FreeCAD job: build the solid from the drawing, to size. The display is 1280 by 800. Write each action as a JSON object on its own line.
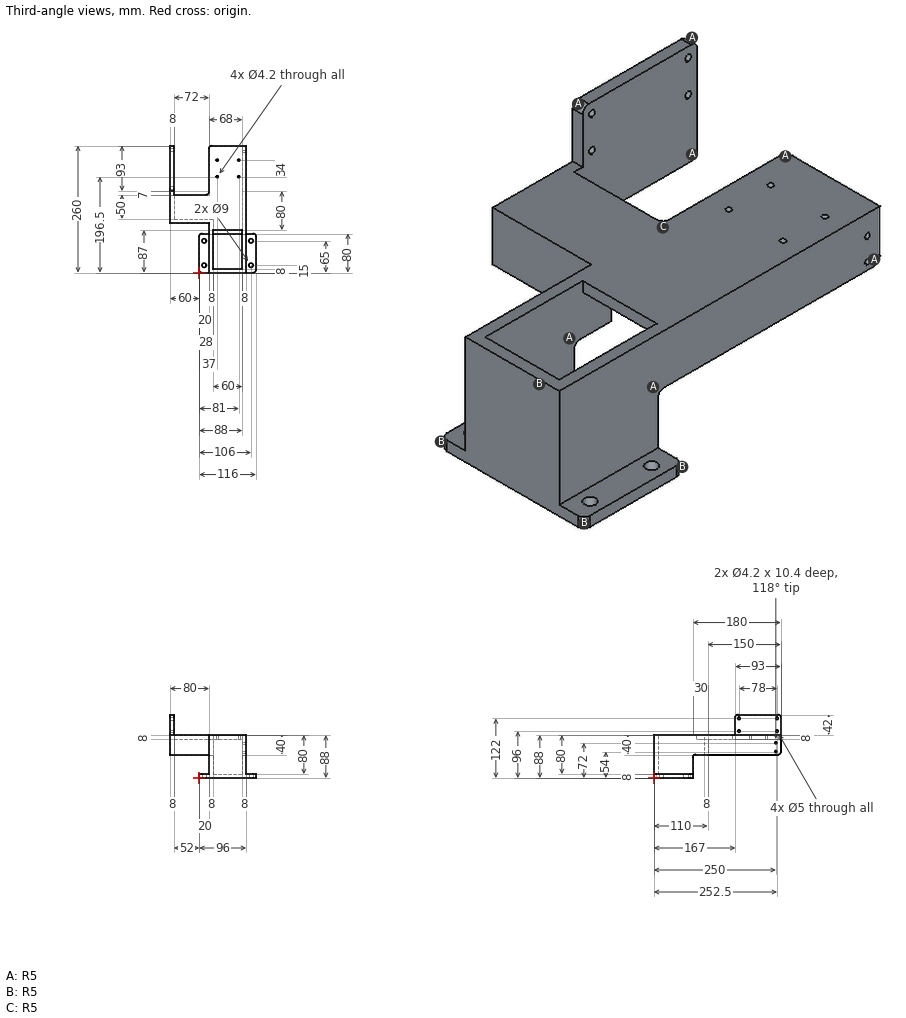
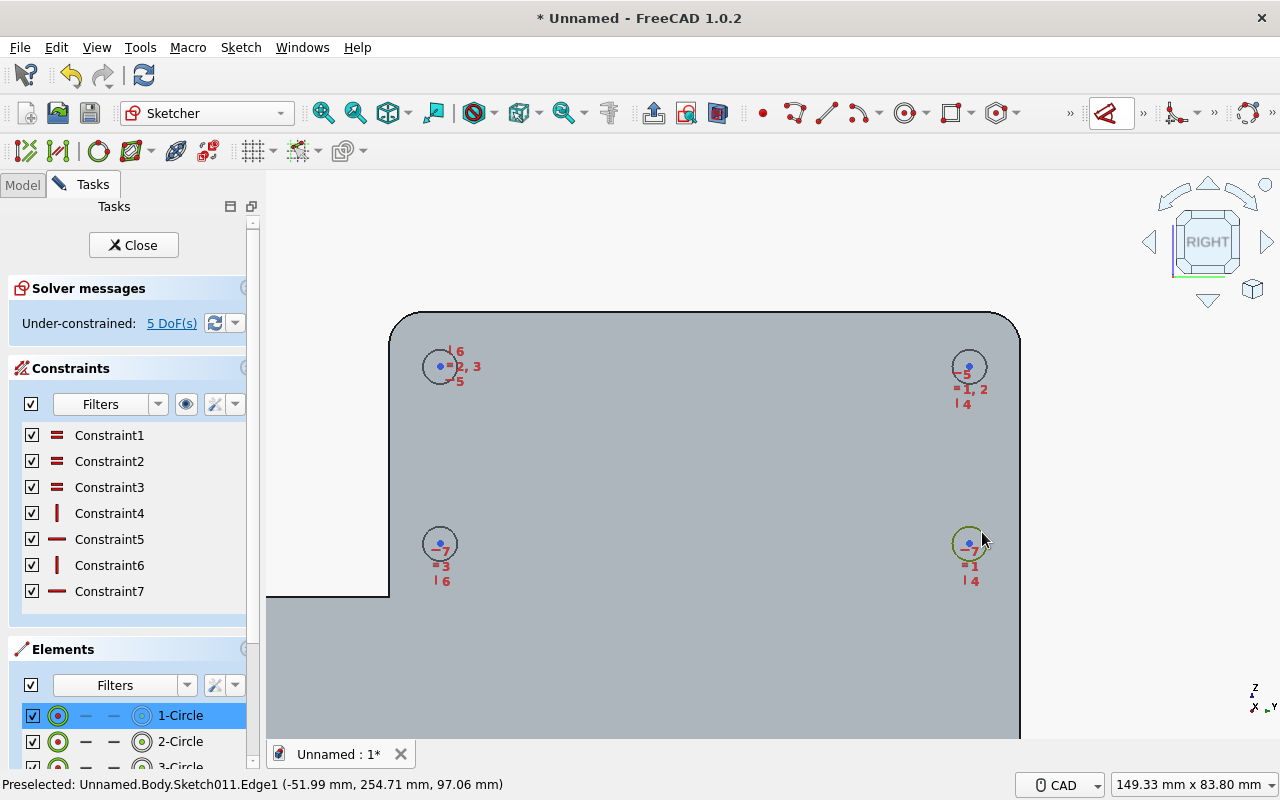
{"action": "left_click", "coordinate": [1128, 114]}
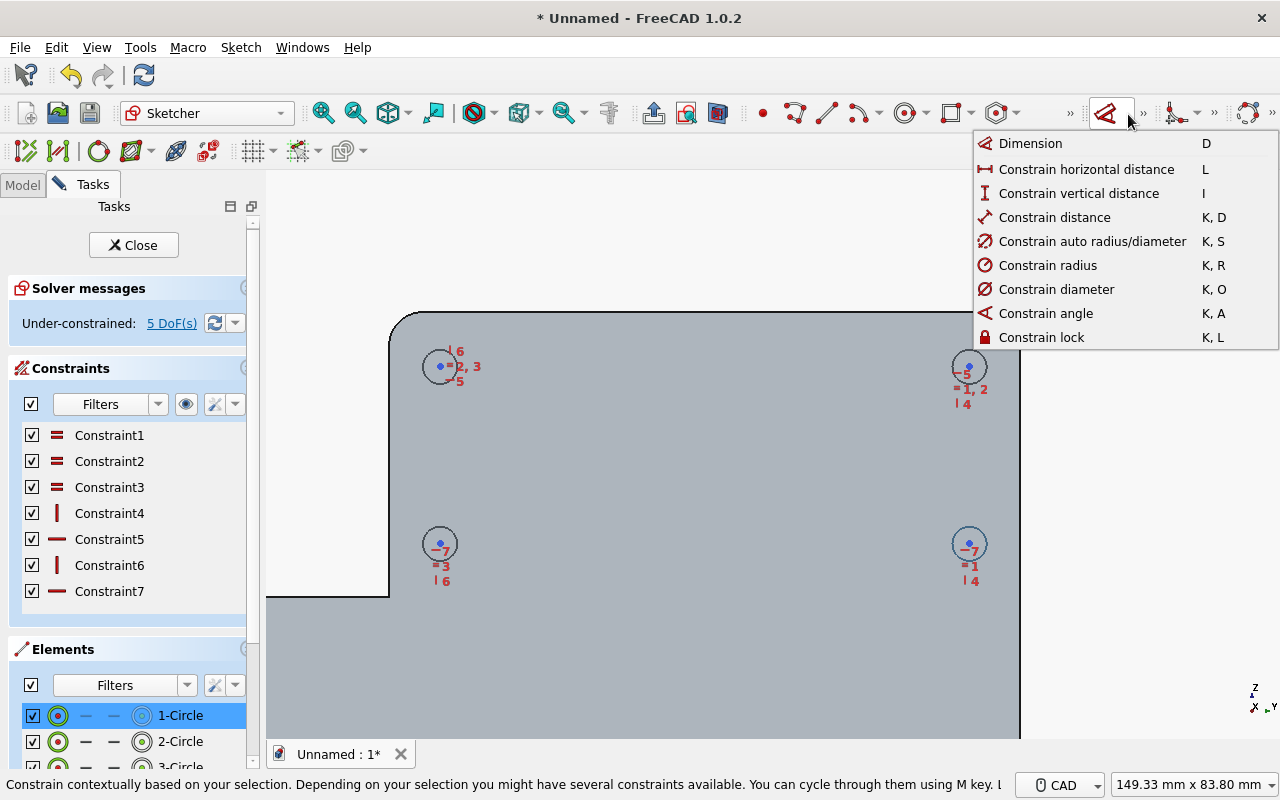
{"action": "left_click", "coordinate": [1126, 289]}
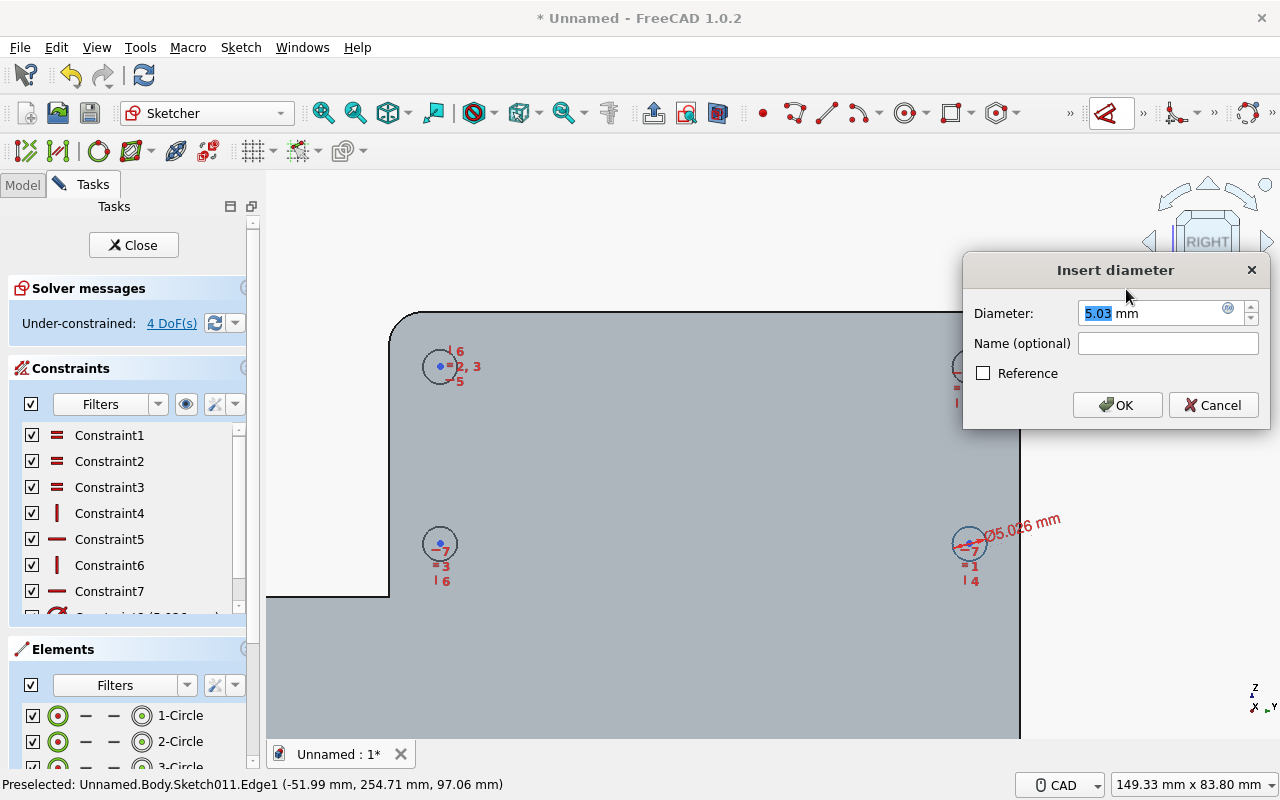
{"action": "type", "text": "5"}
{"action": "key", "text": "Return"}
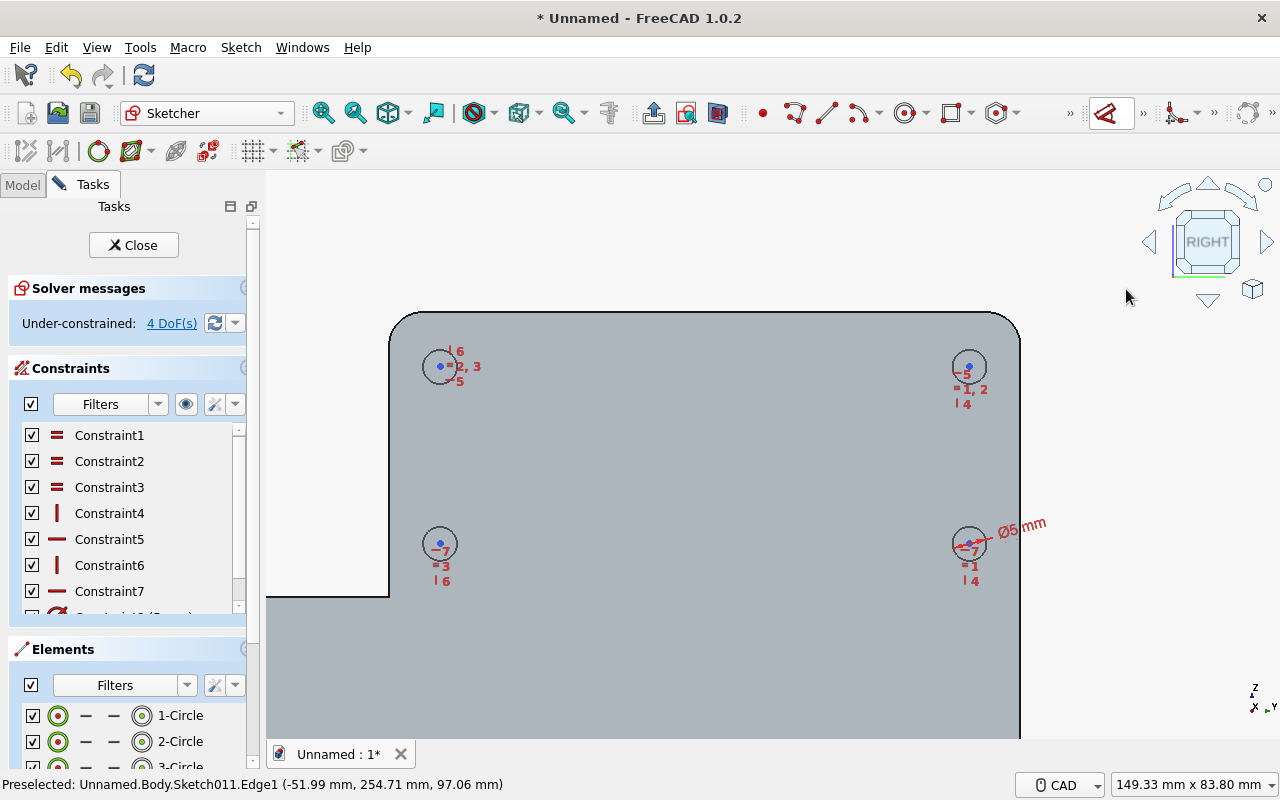
{"action": "left_click", "coordinate": [970, 544]}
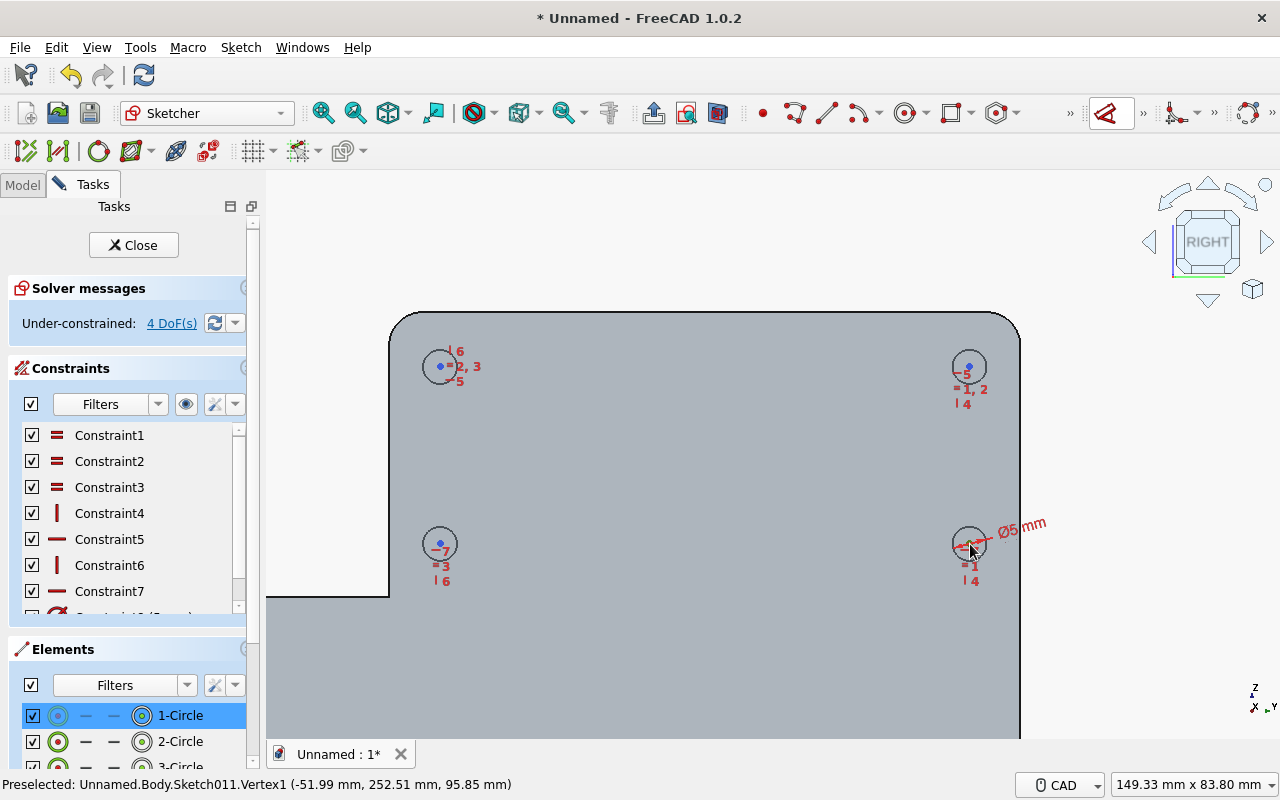
{"action": "left_click", "coordinate": [1128, 114]}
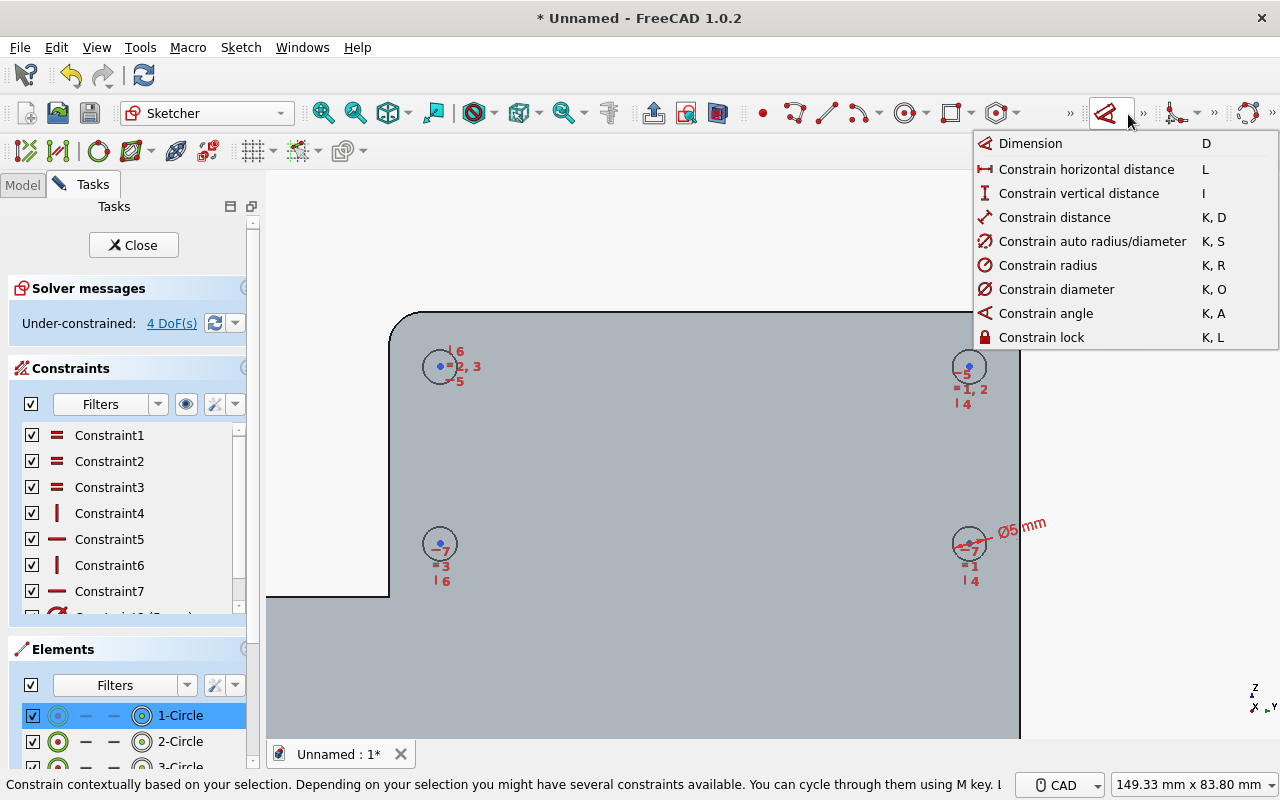
{"action": "left_click", "coordinate": [1126, 193]}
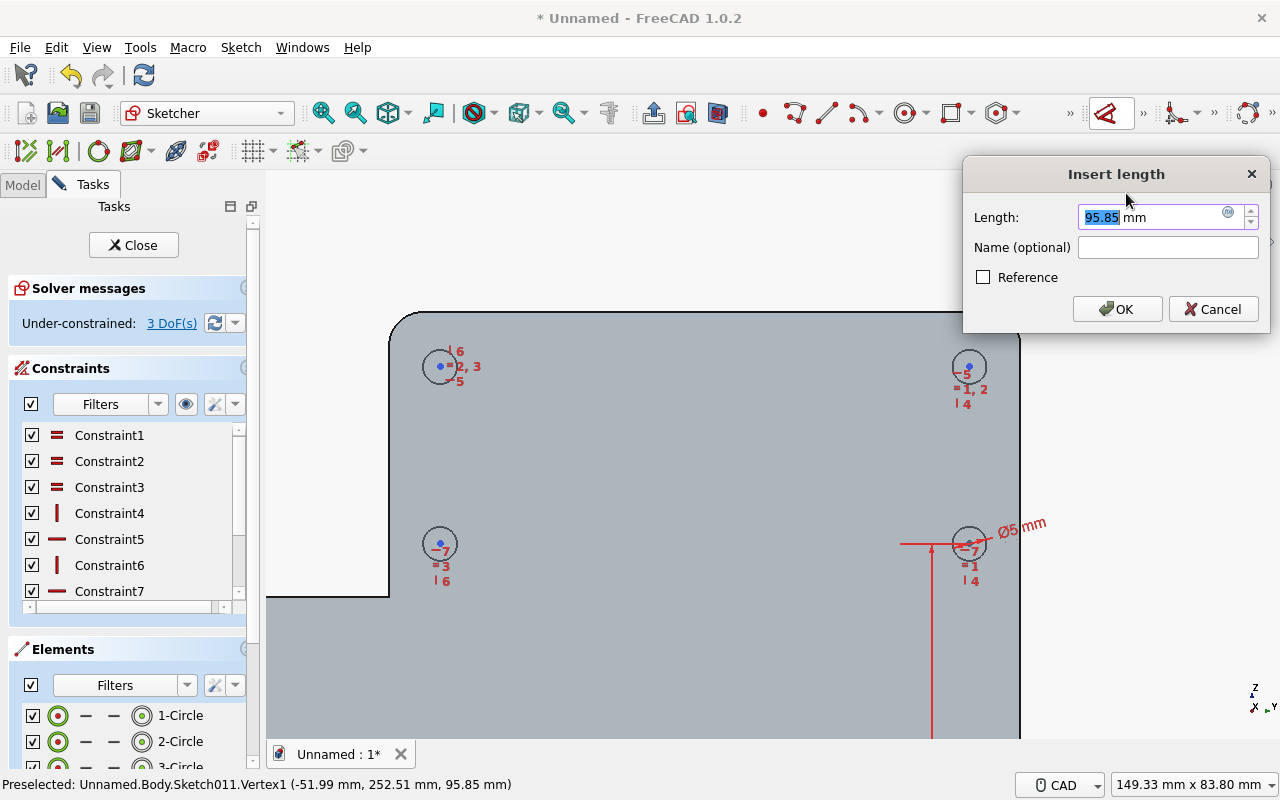
{"action": "type", "text": "96"}
{"action": "key", "text": "Return"}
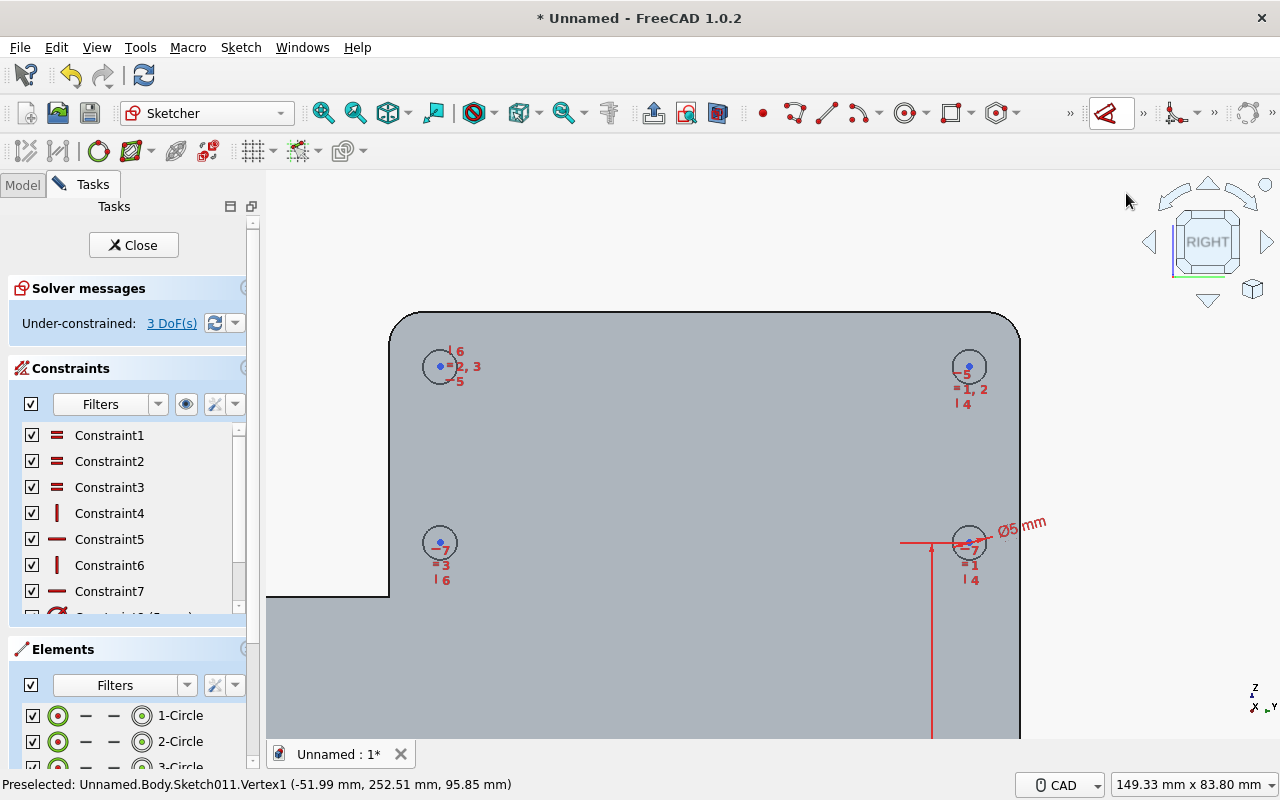
{"action": "left_click", "coordinate": [970, 367]}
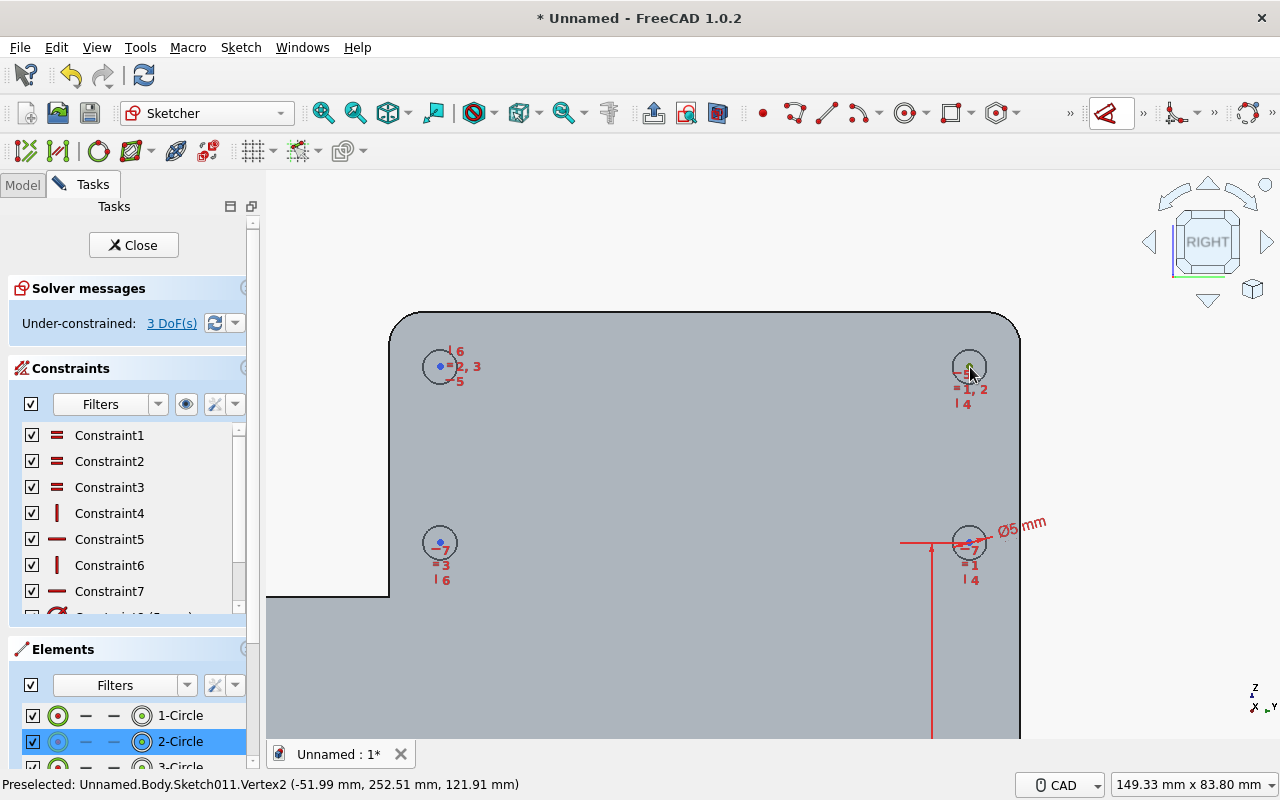
{"action": "left_click", "coordinate": [1128, 114]}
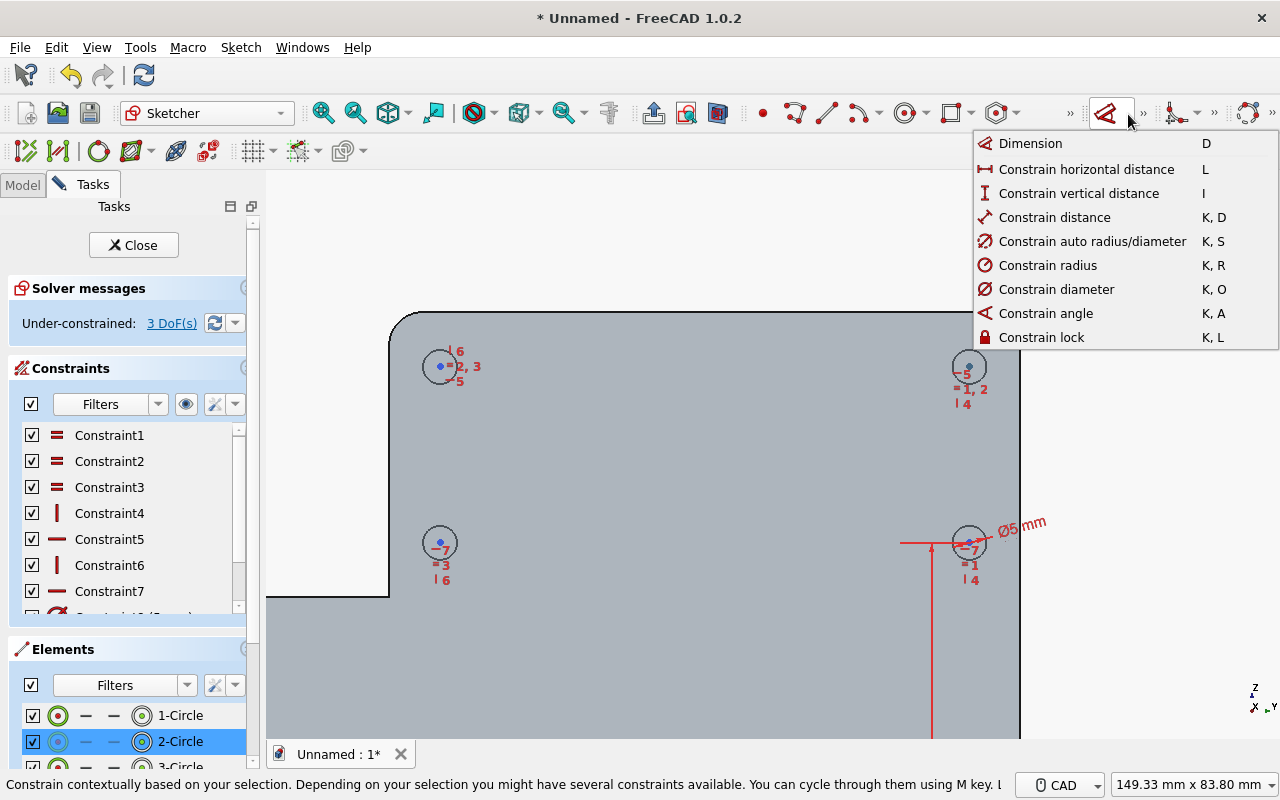
{"action": "left_click", "coordinate": [1126, 193]}